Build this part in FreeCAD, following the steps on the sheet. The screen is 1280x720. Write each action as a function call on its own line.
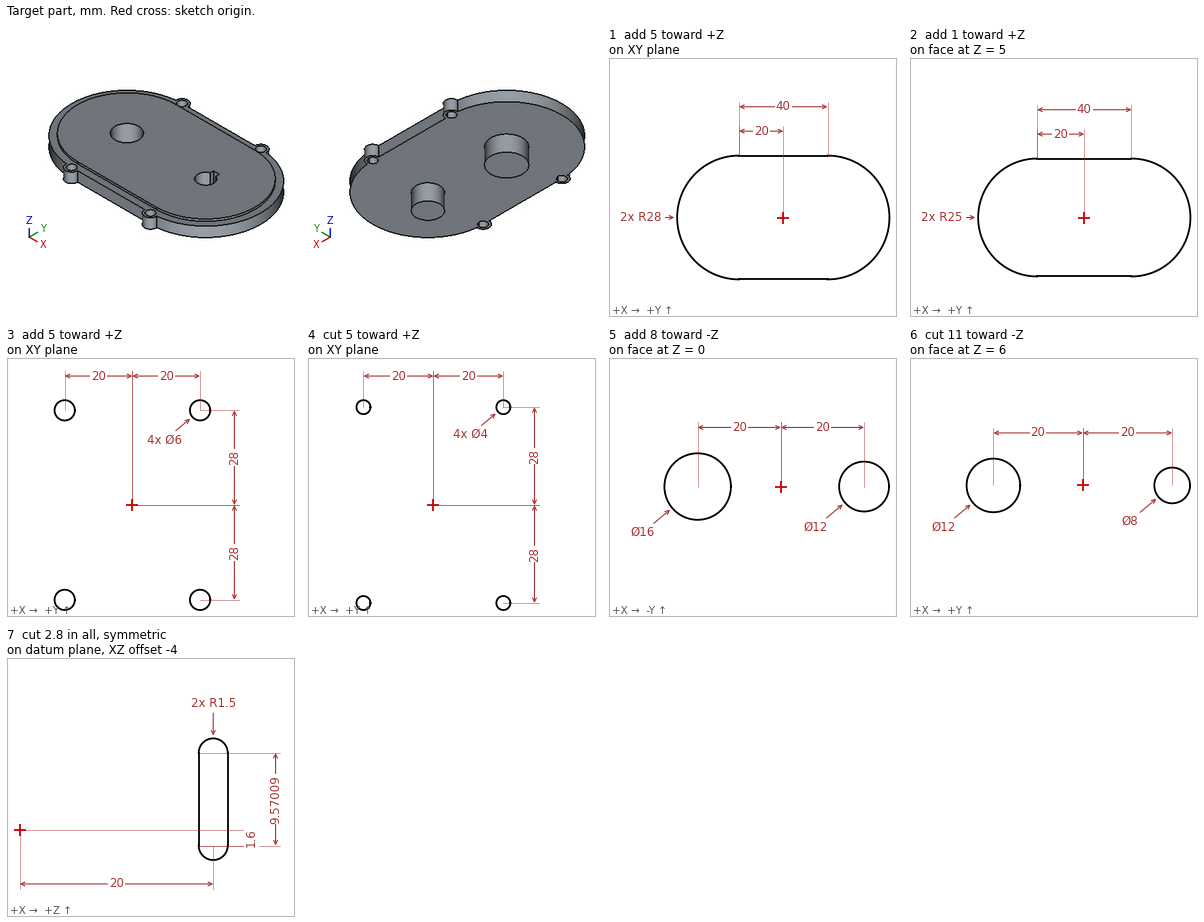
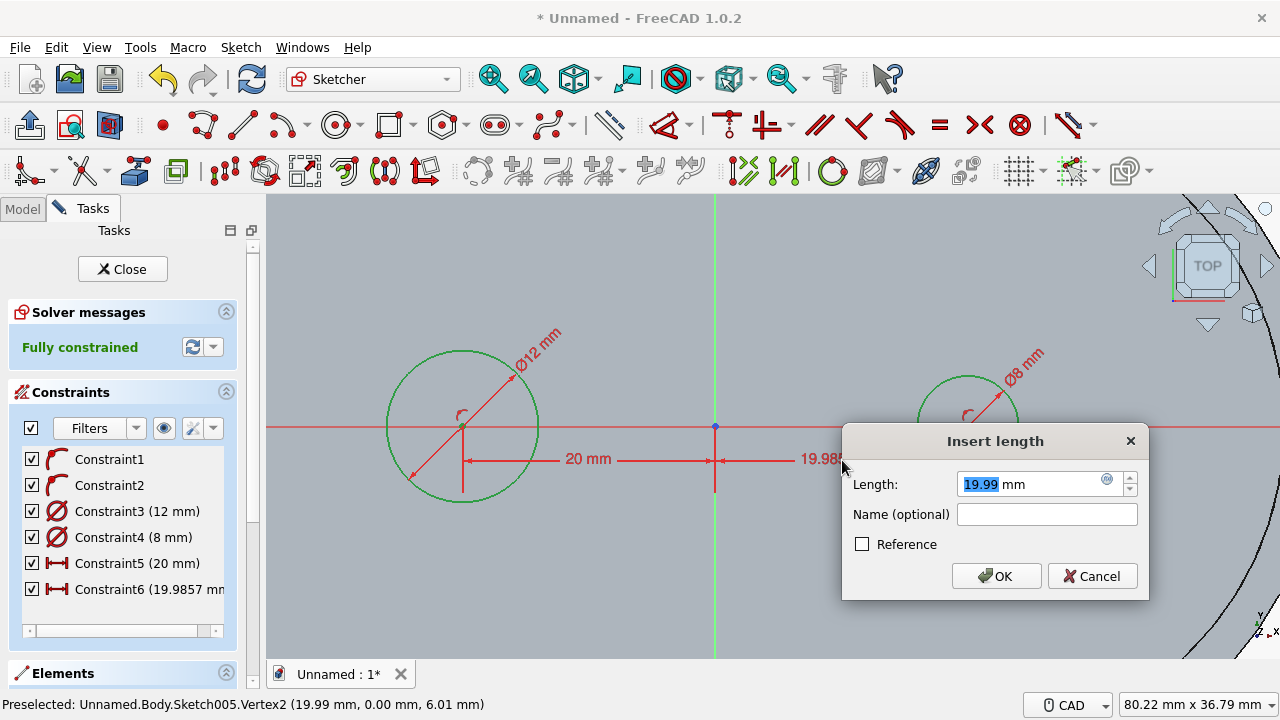
text(20)
key(Return)
key(Escape)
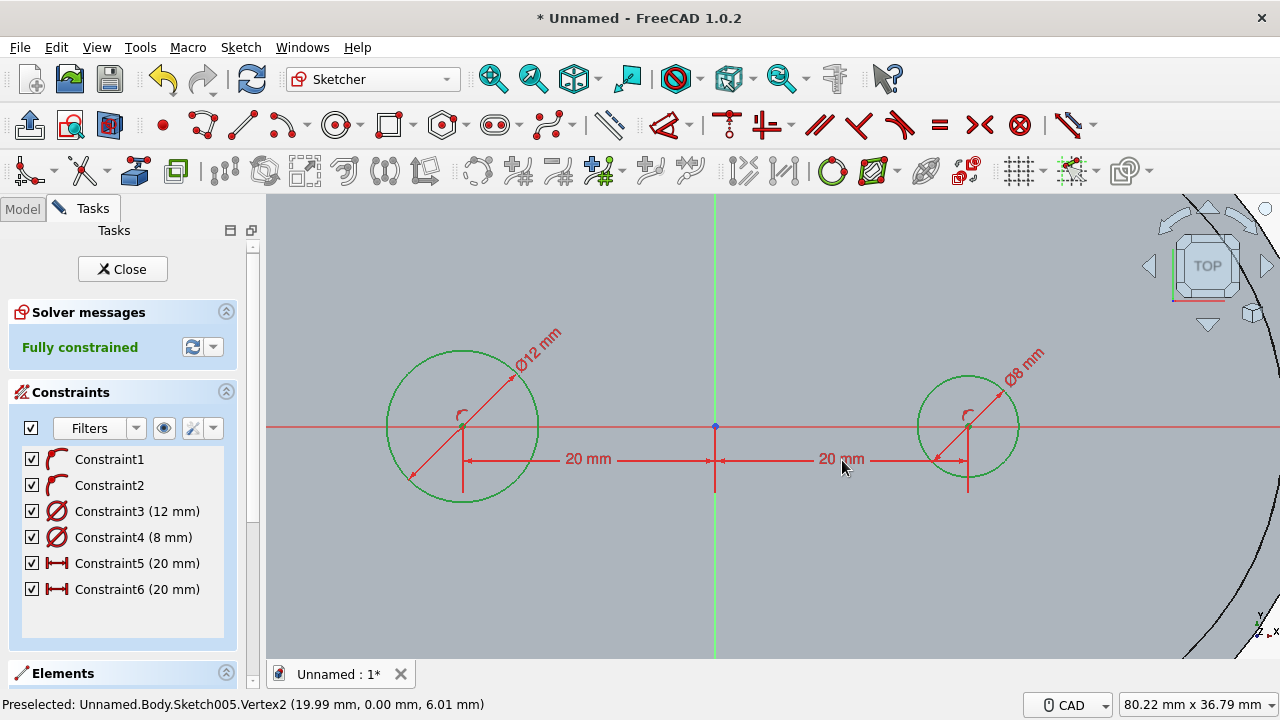
click(123, 269)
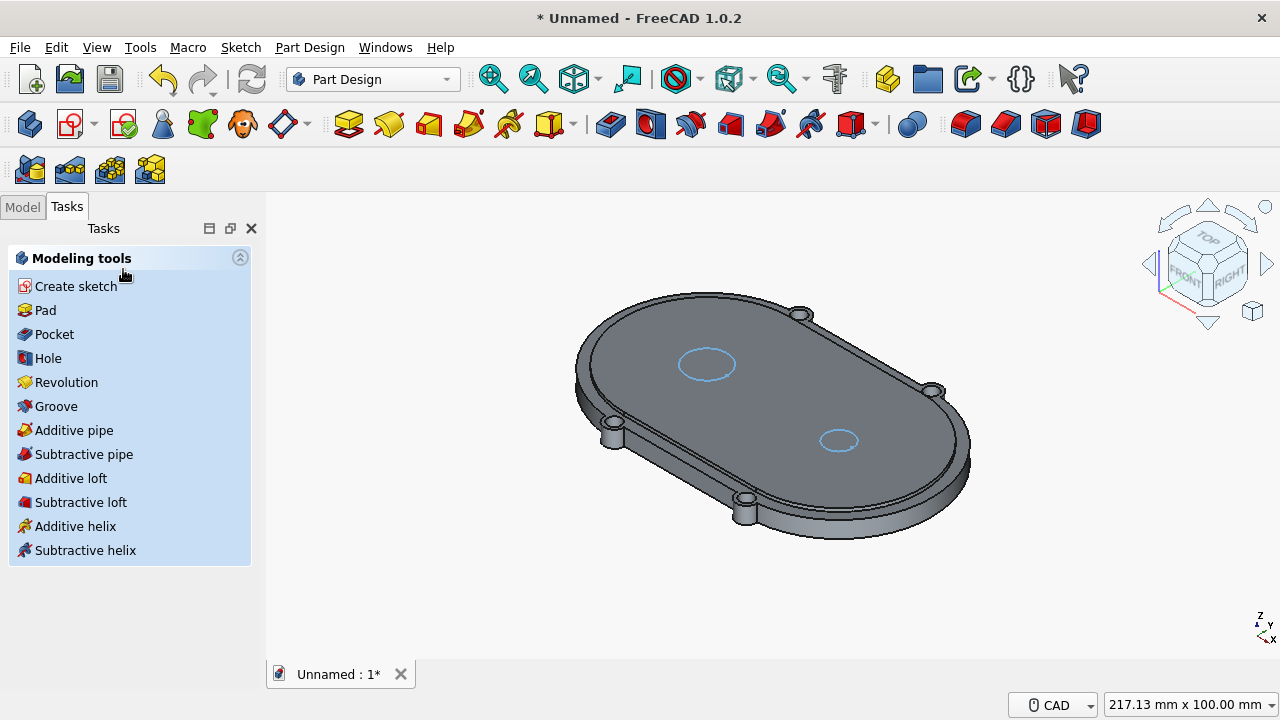
click(612, 124)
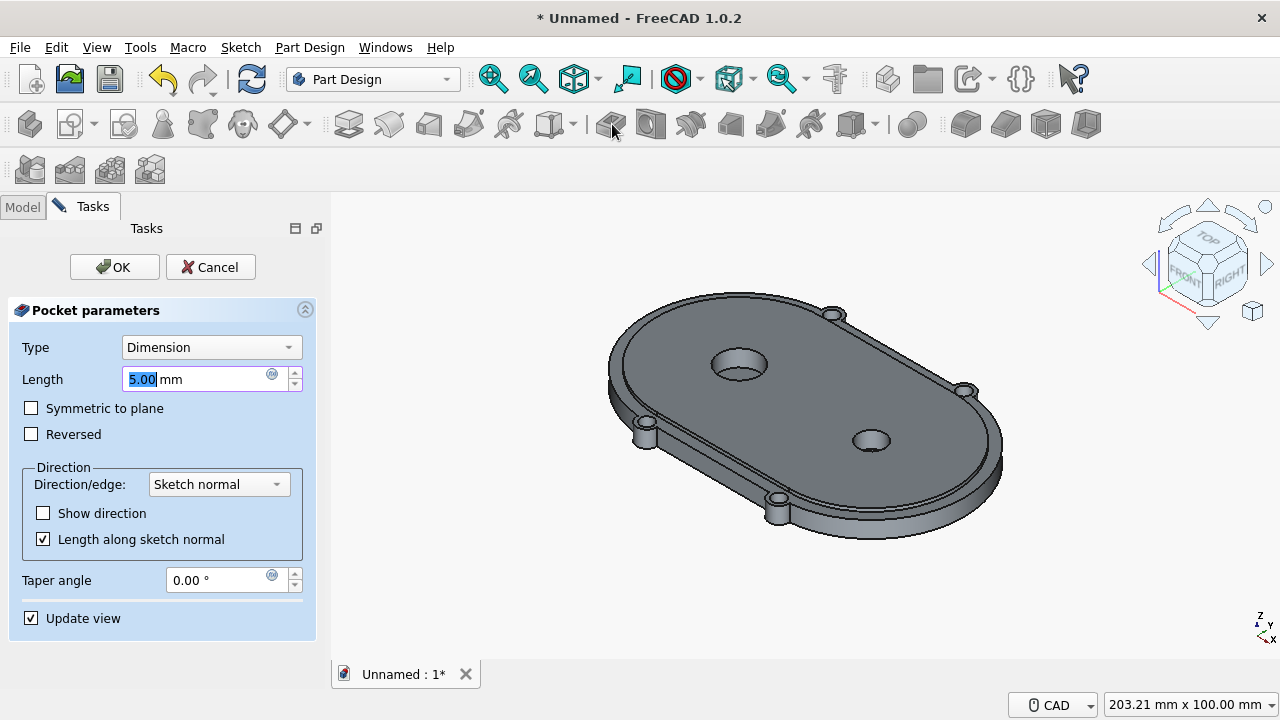
text(11)
key(Tab)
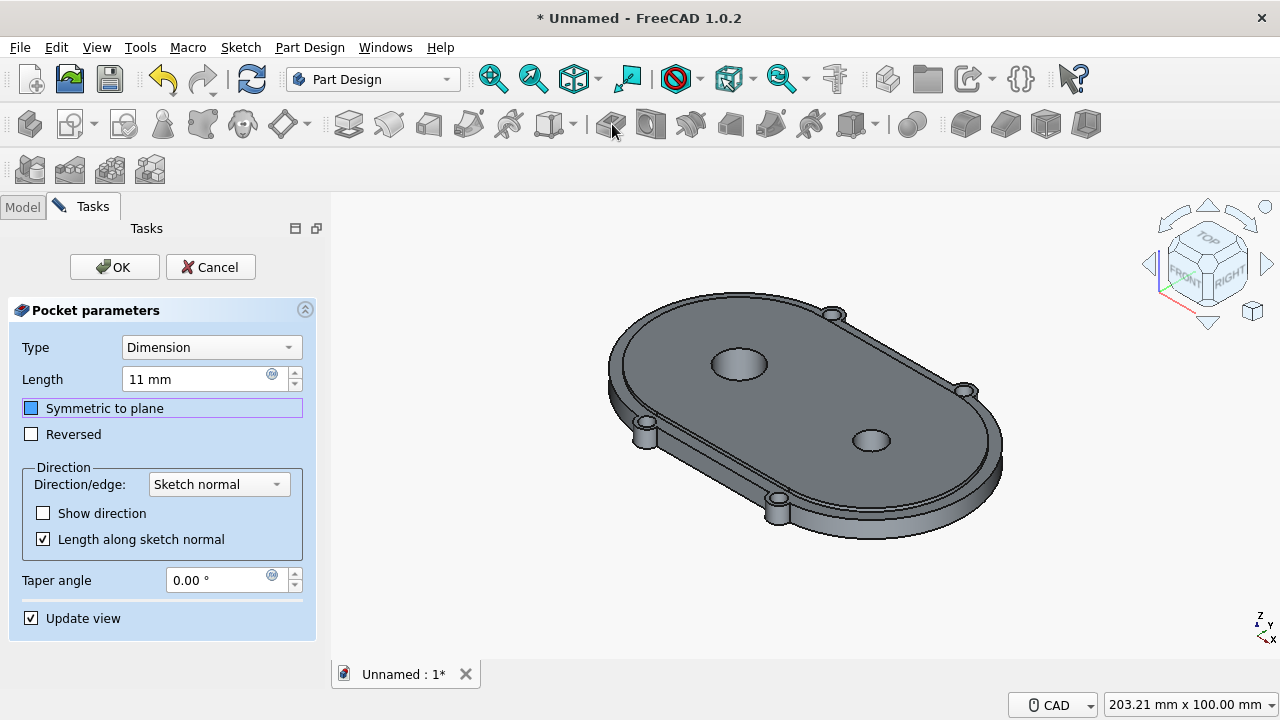
click(115, 267)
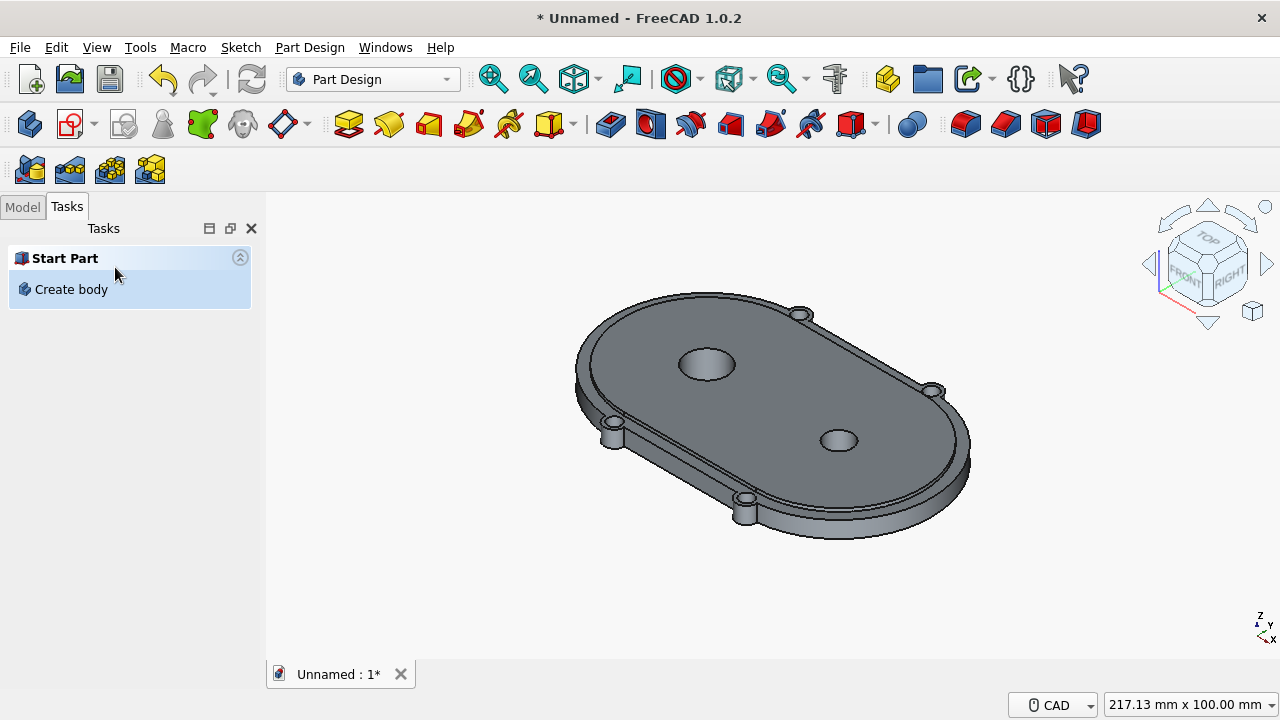
click(23, 206)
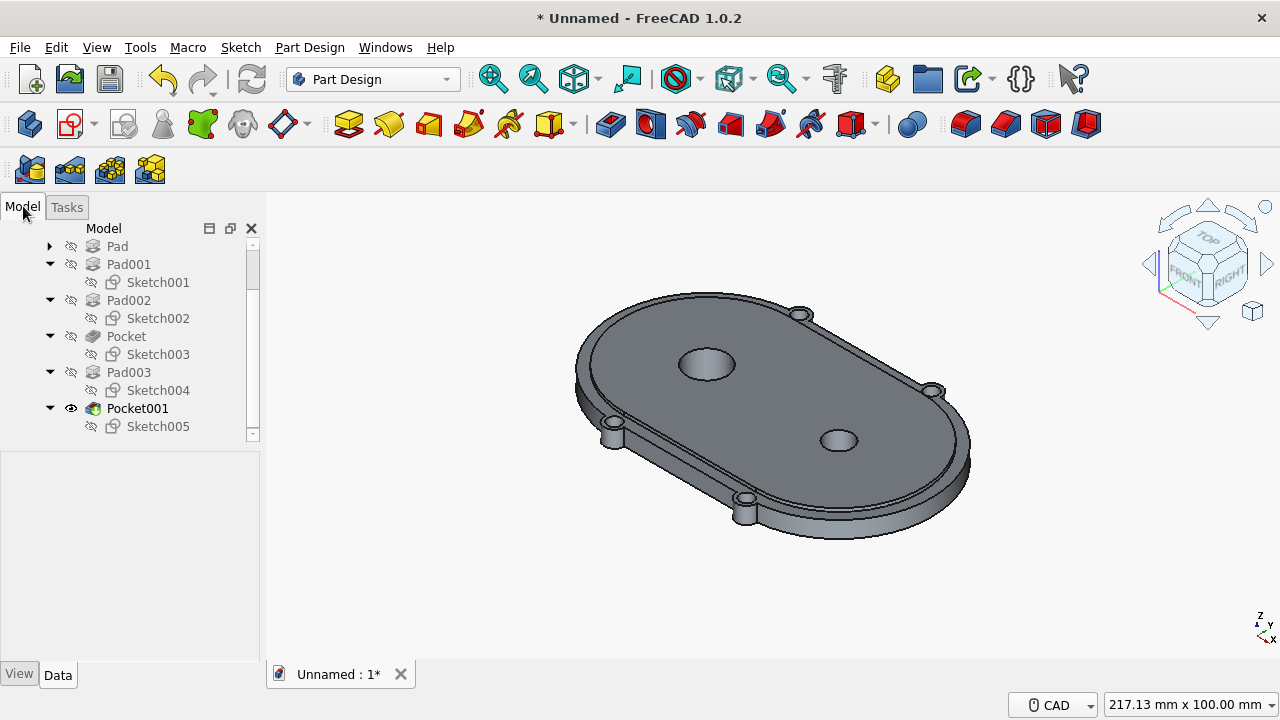
scroll(140, 332, down, 3)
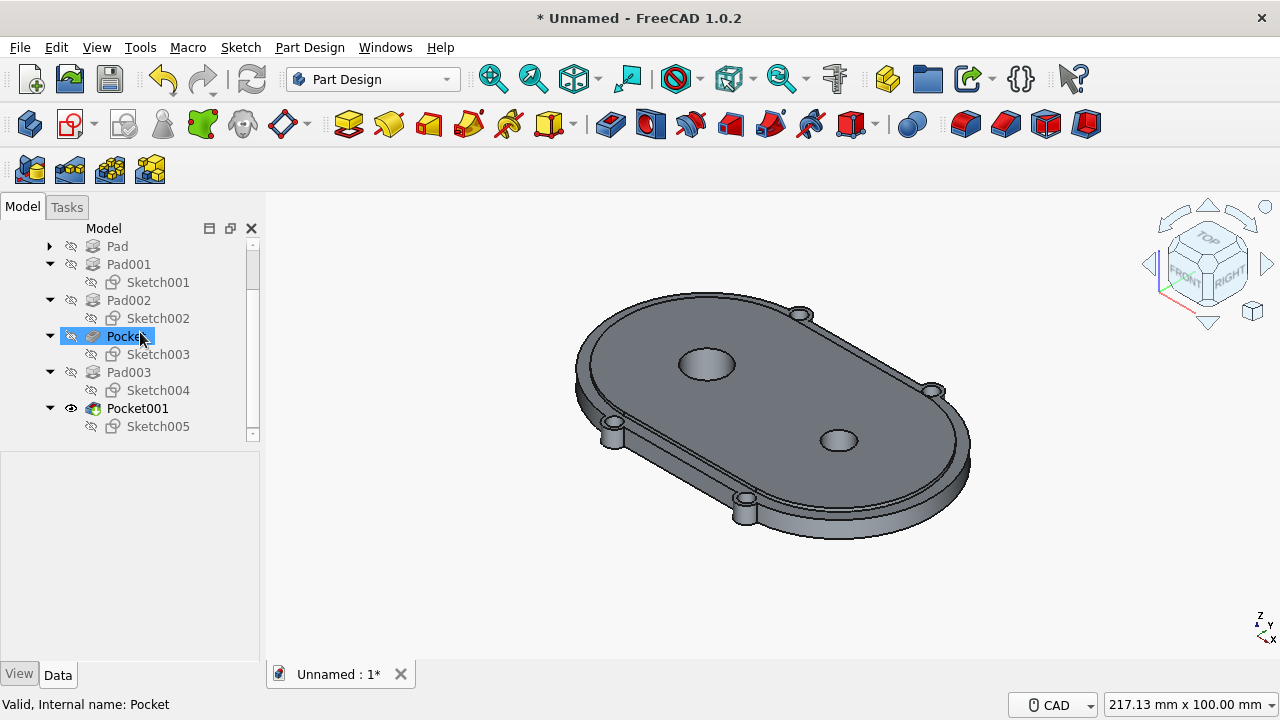
scroll(140, 332, up, 15)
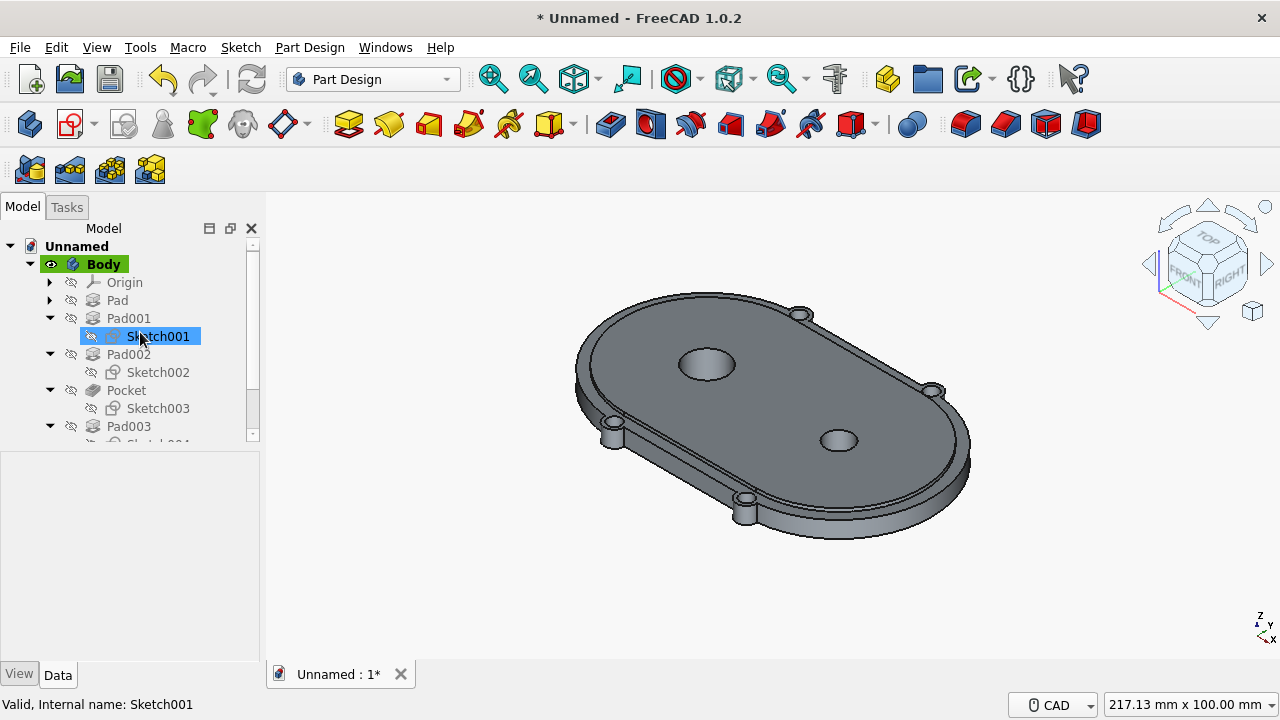
click(50, 282)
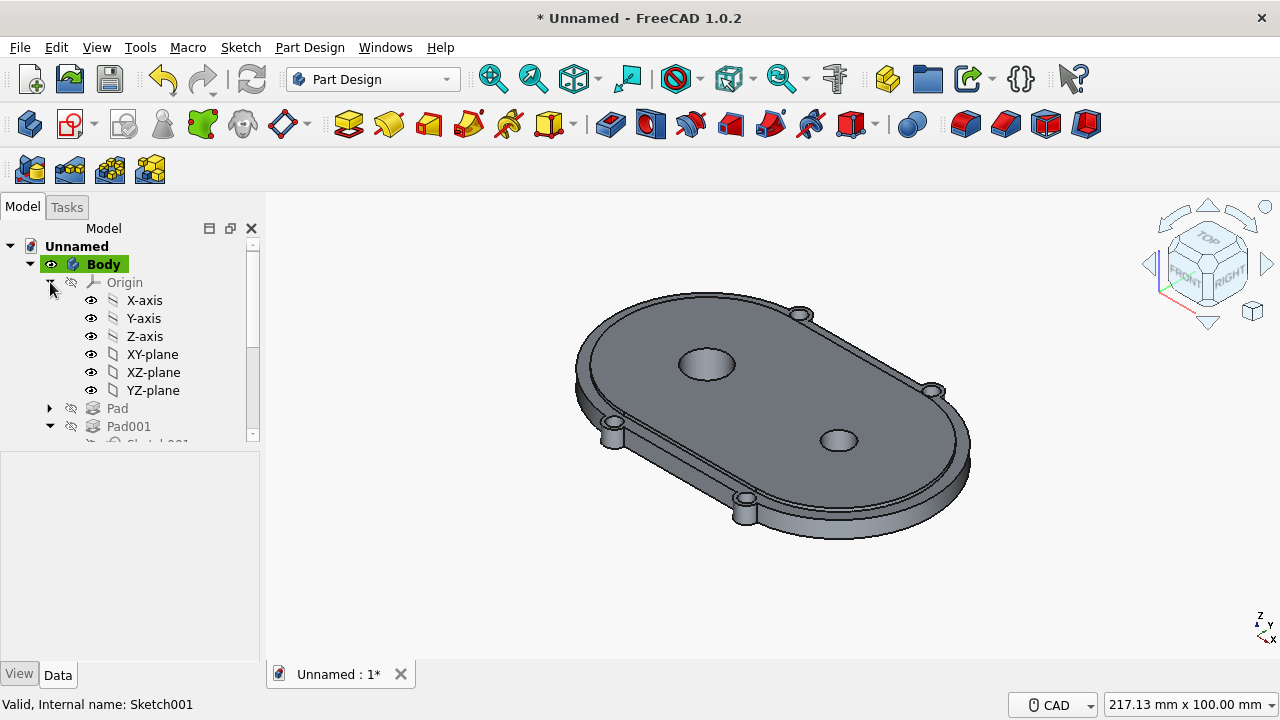
click(136, 372)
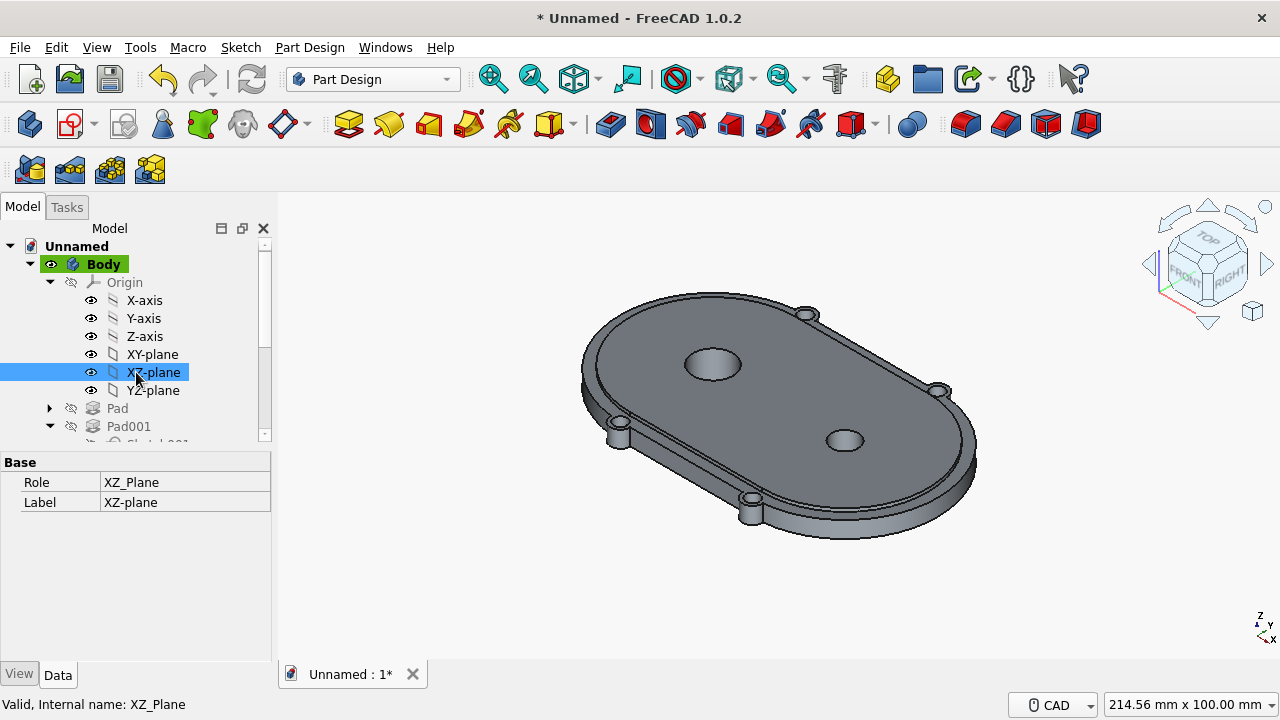
click(284, 124)